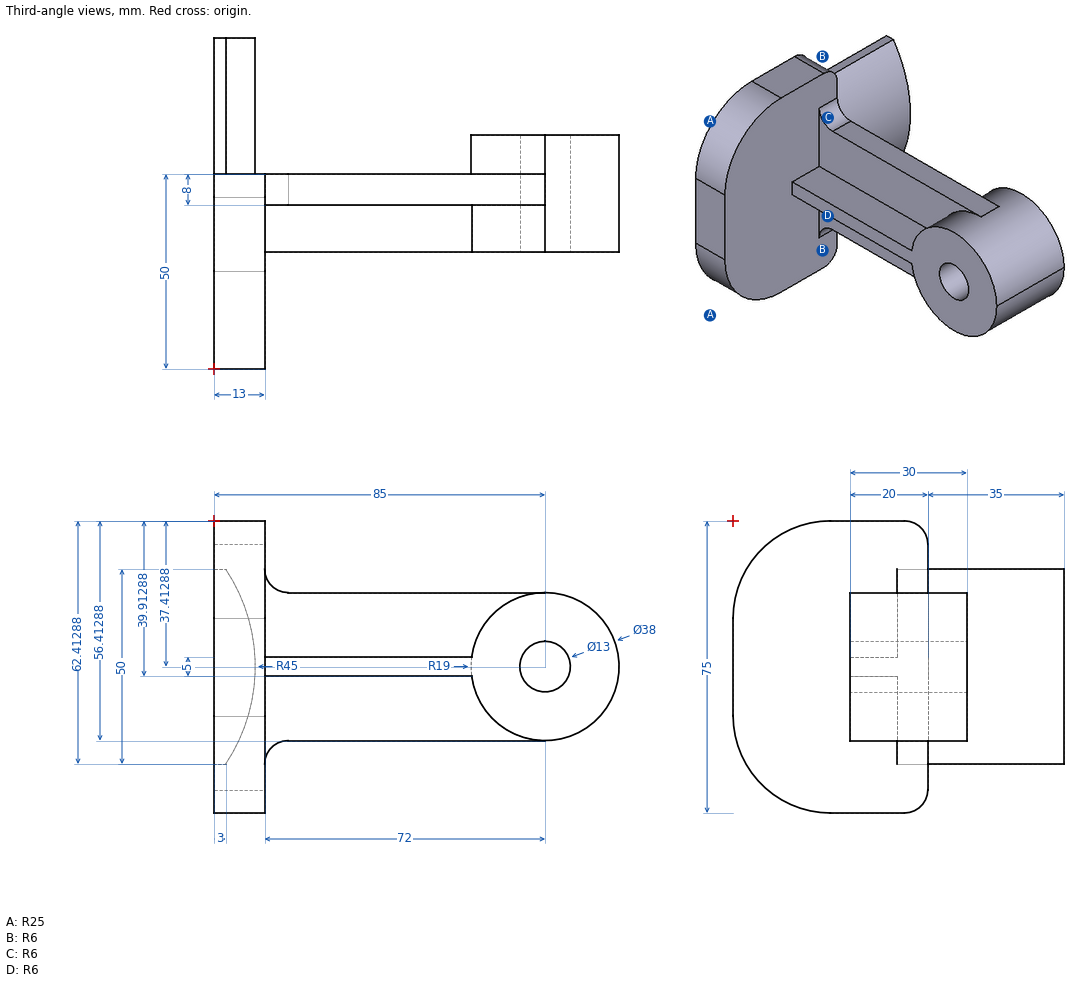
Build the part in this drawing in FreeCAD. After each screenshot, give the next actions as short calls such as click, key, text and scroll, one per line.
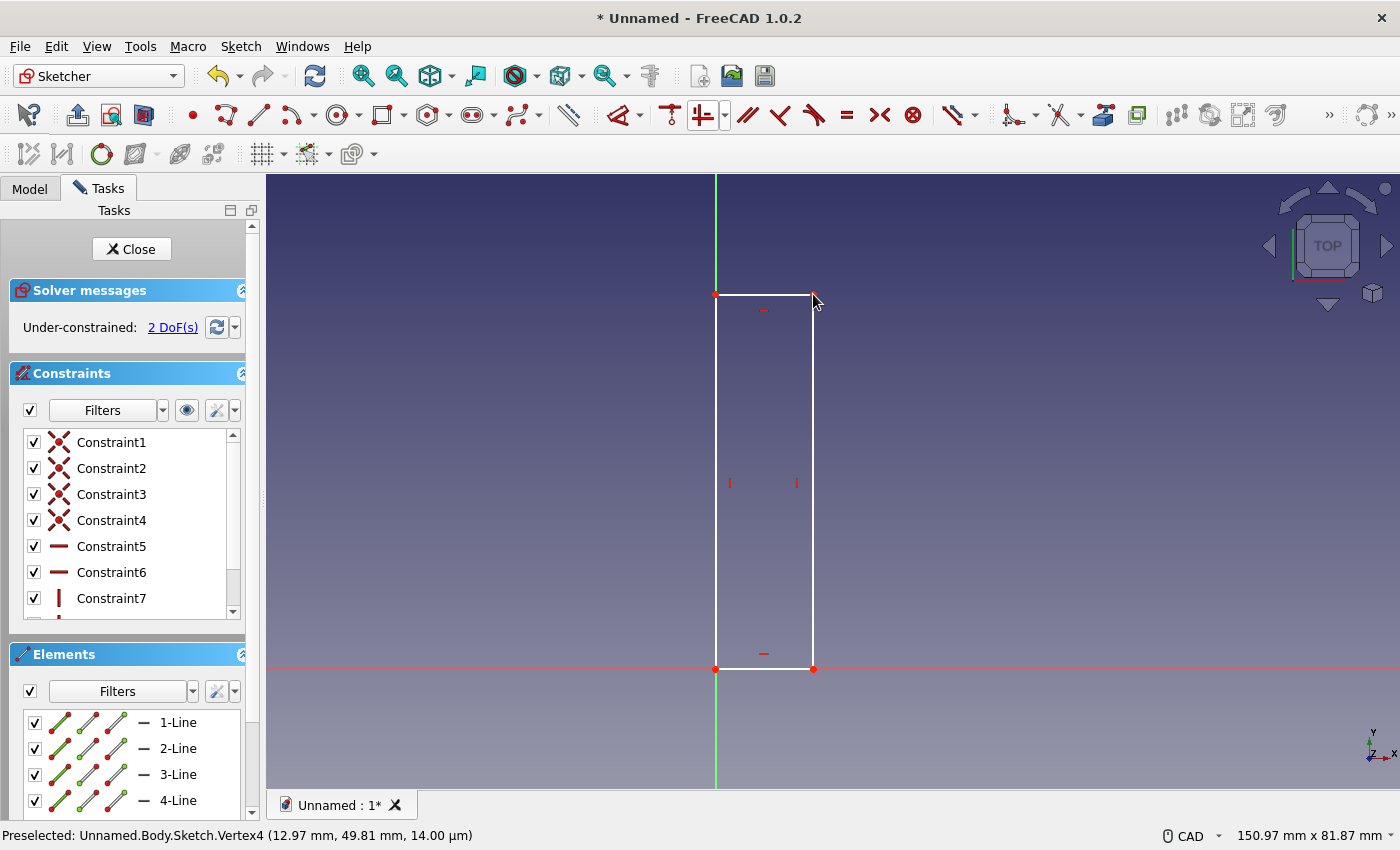
click(618, 116)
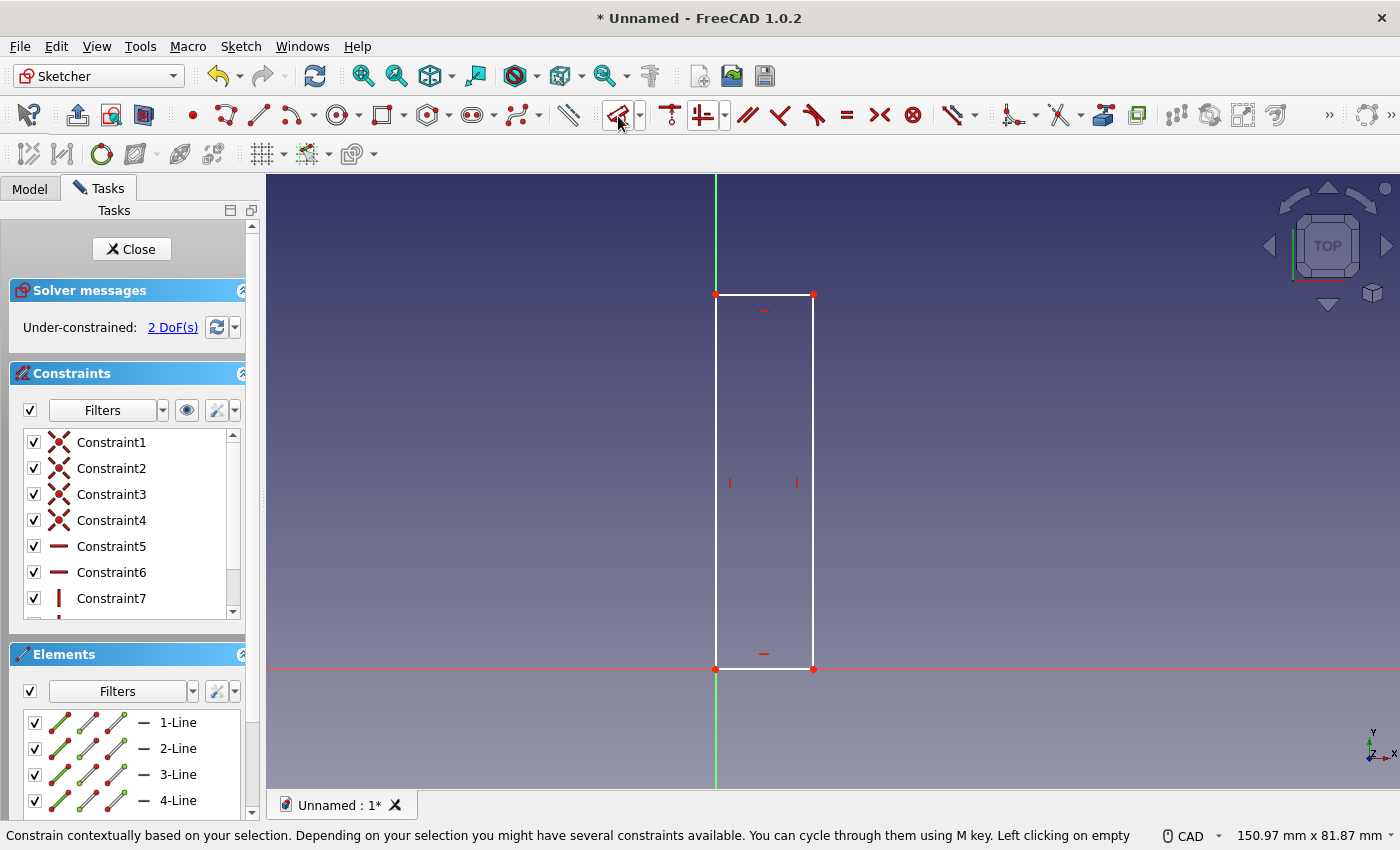
click(745, 669)
click(764, 703)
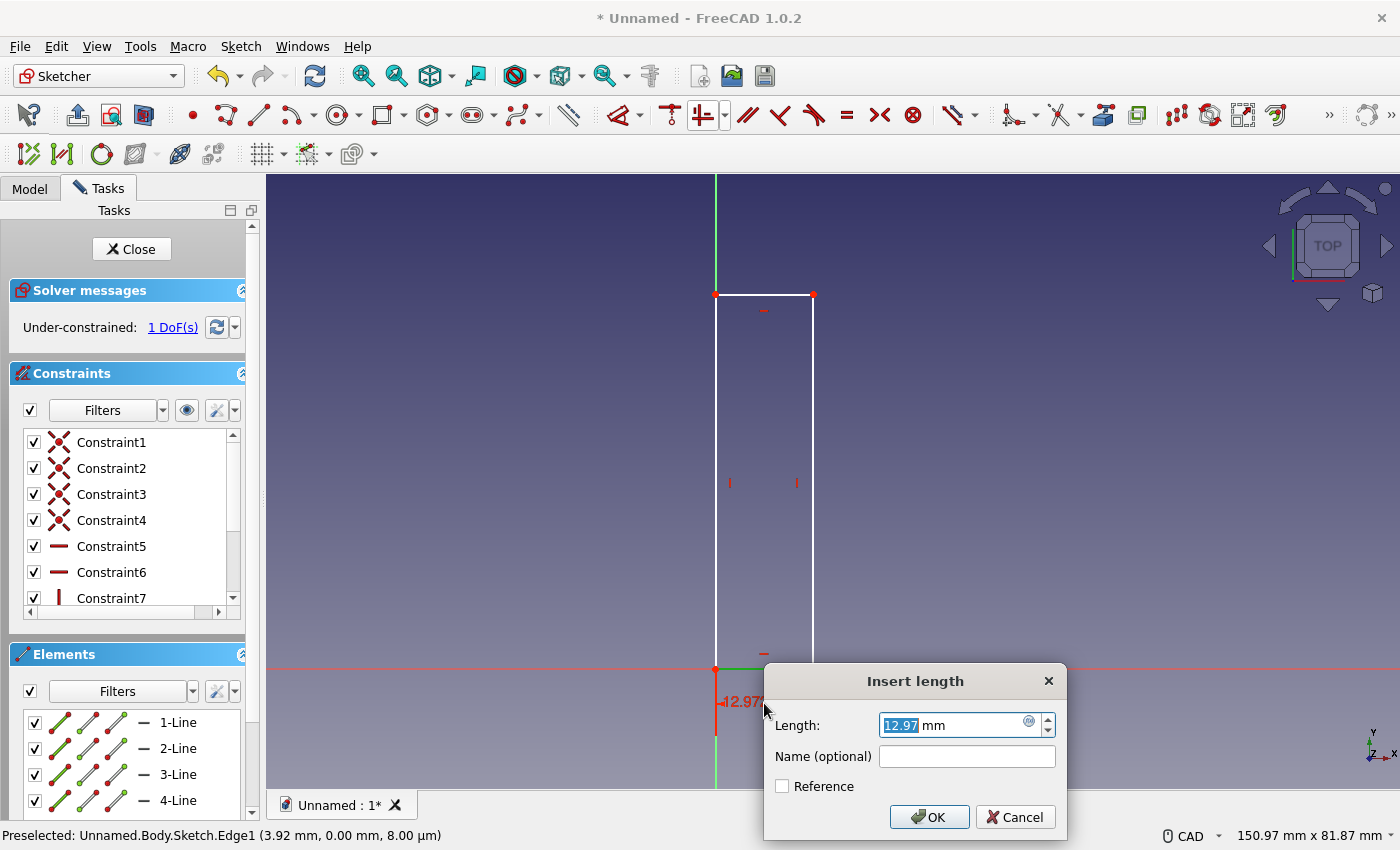
text(13)
key(Return)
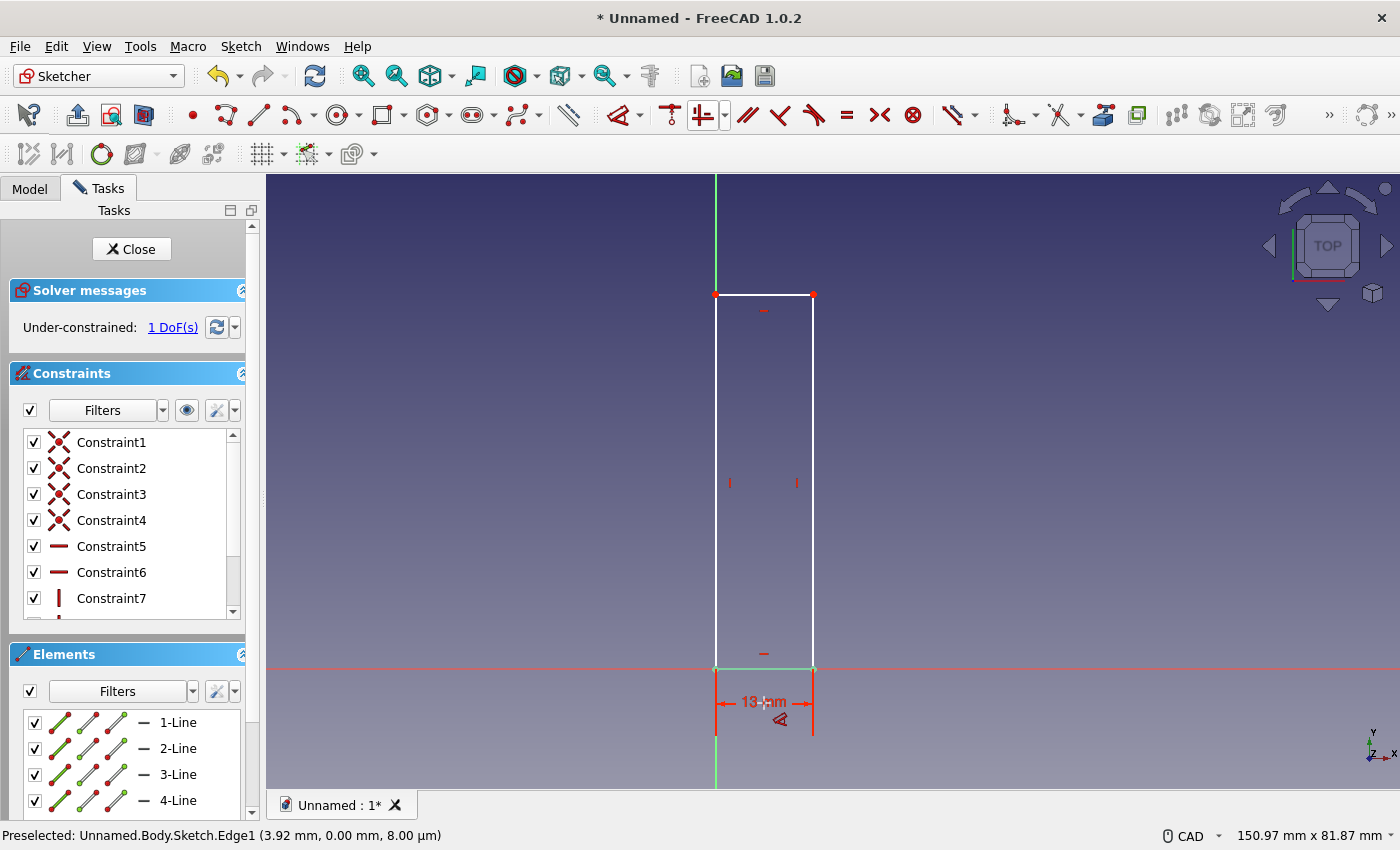
click(813, 557)
click(847, 482)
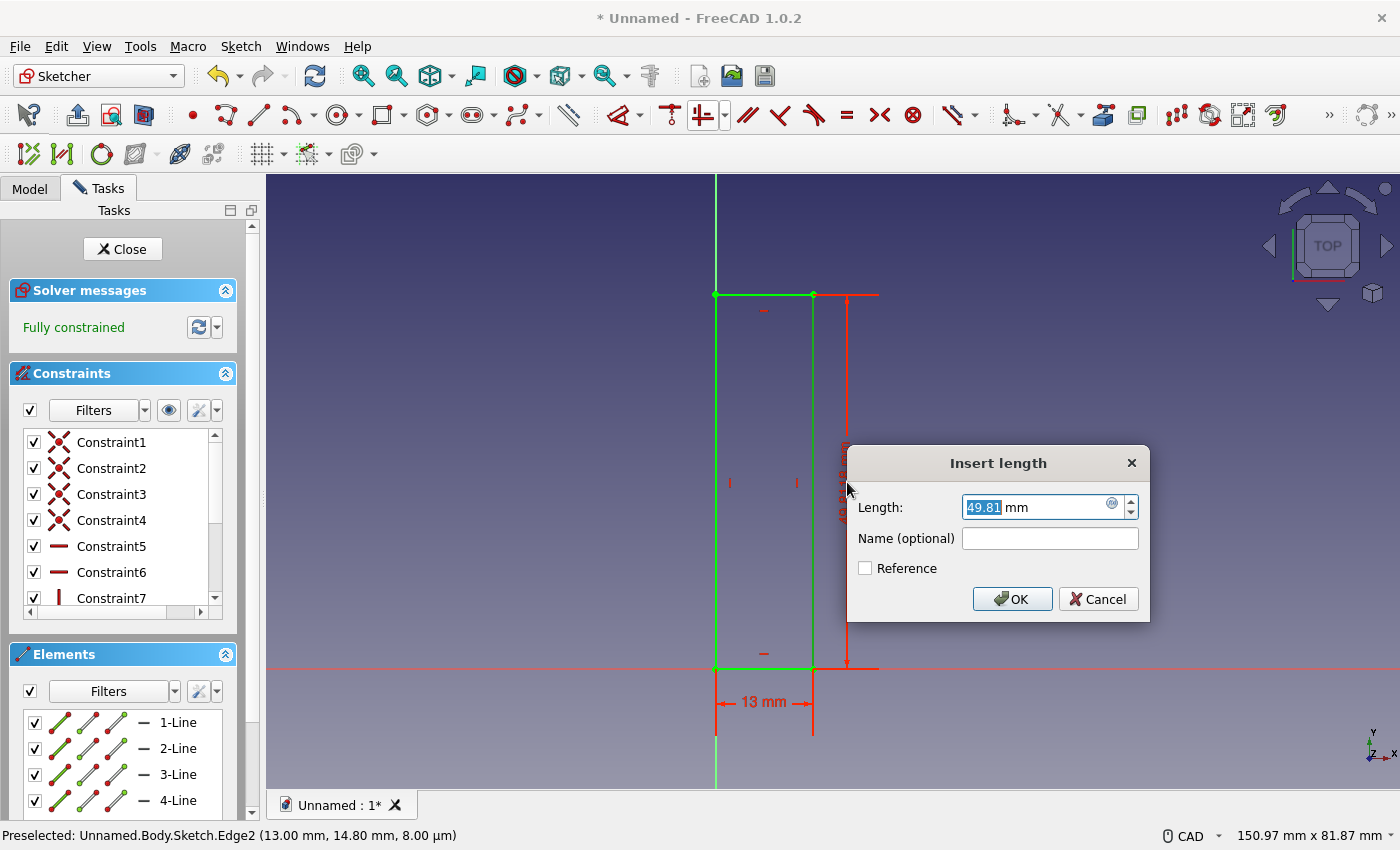
text(50)
key(Return)
key(Escape)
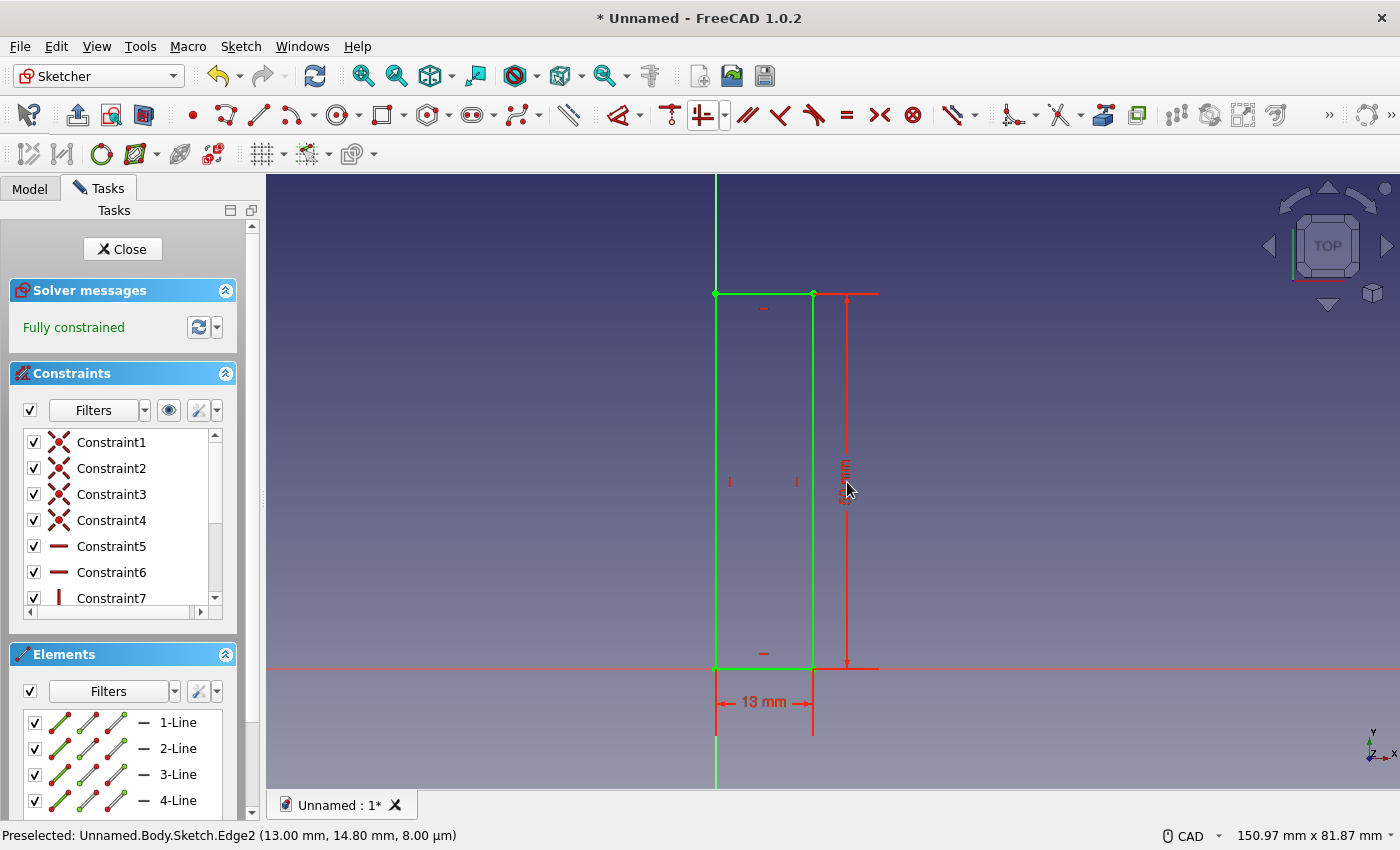
click(123, 249)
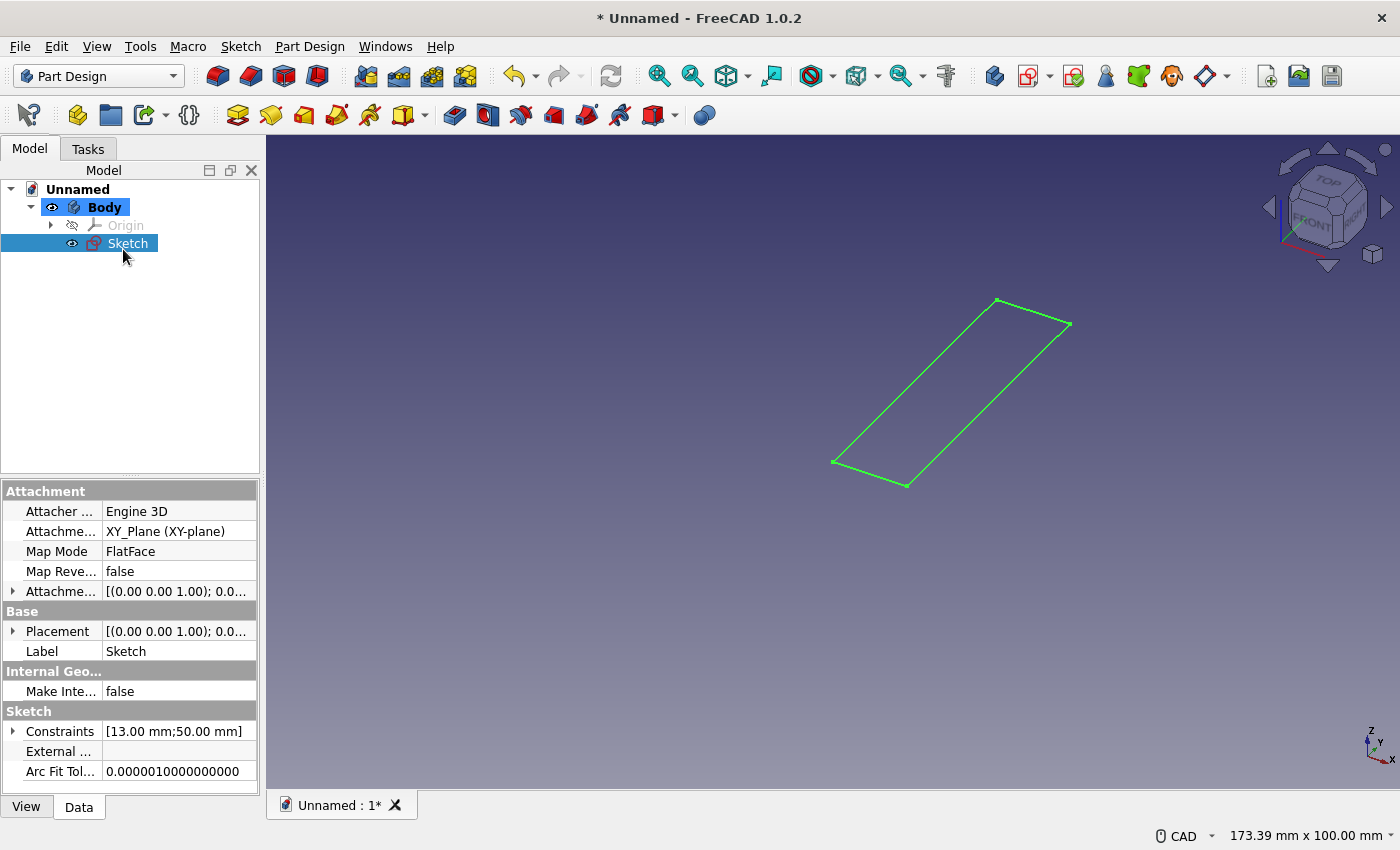
click(238, 116)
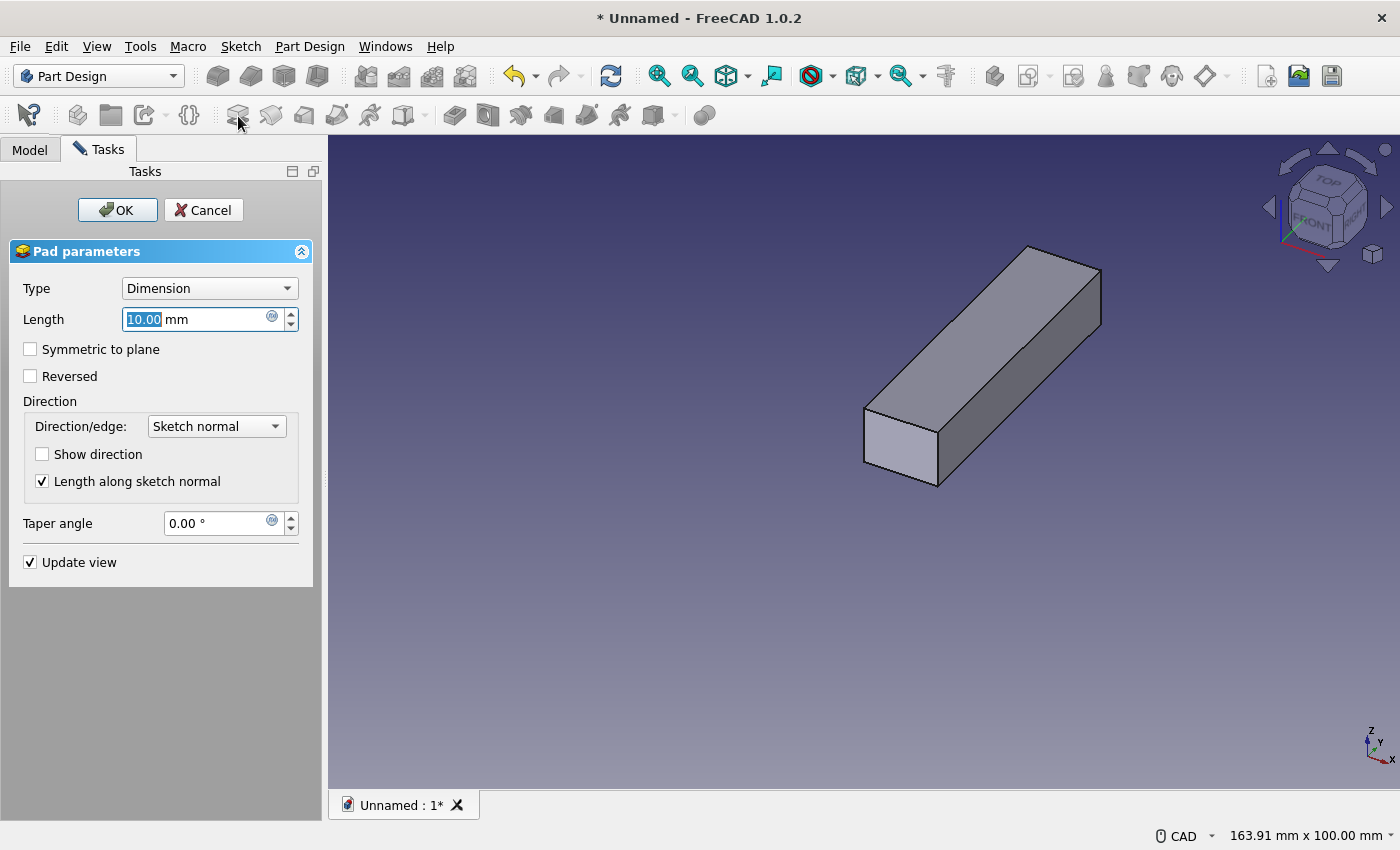
text(75)
key(Tab)